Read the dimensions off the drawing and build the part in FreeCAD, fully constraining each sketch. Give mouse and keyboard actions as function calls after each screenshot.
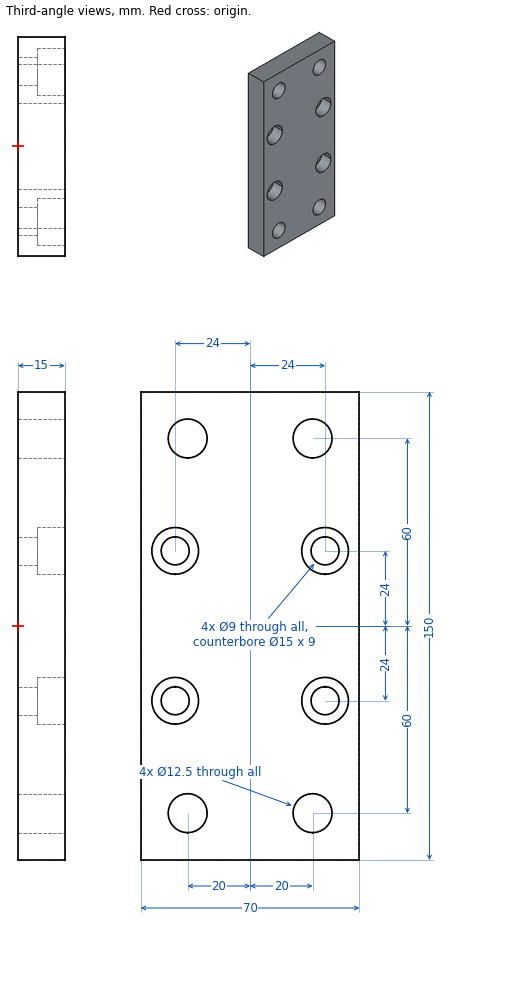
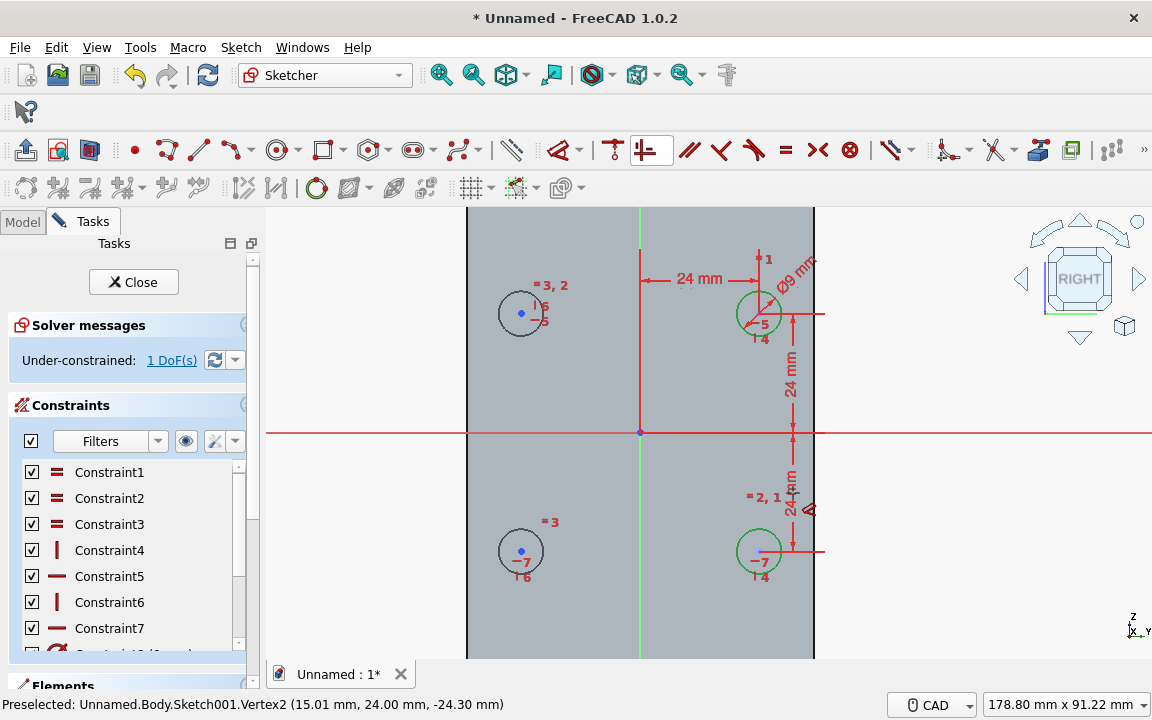
click(521, 314)
click(581, 280)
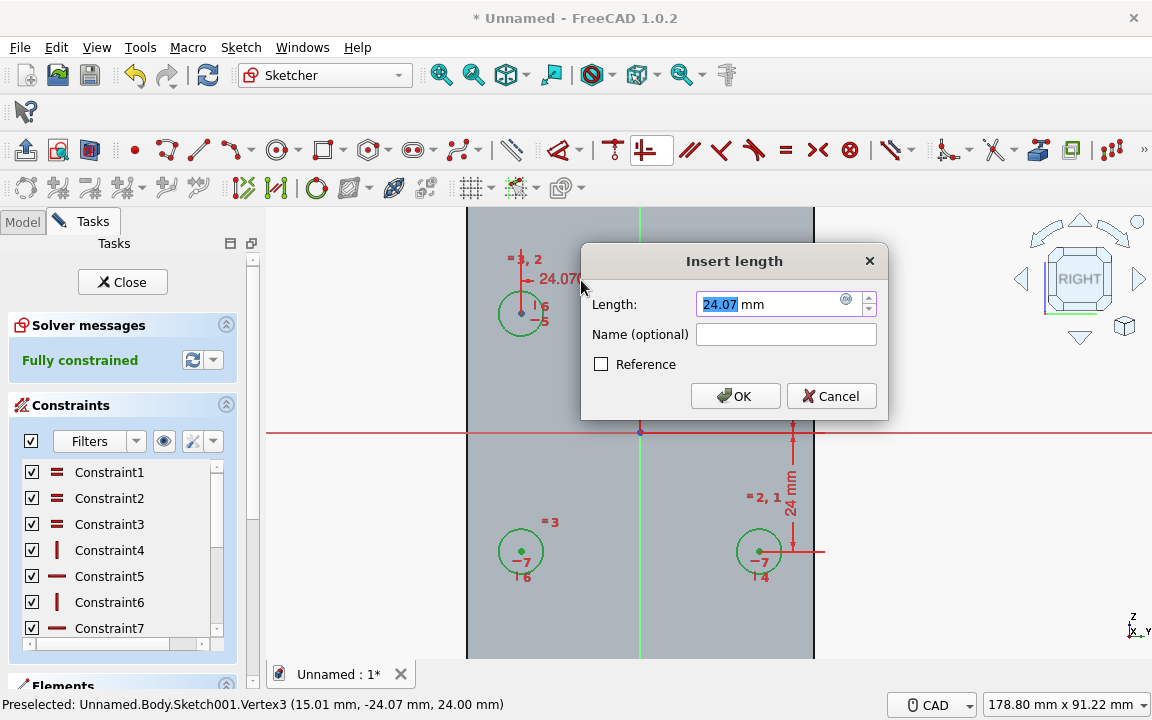
text(24)
key(Return)
key(Escape)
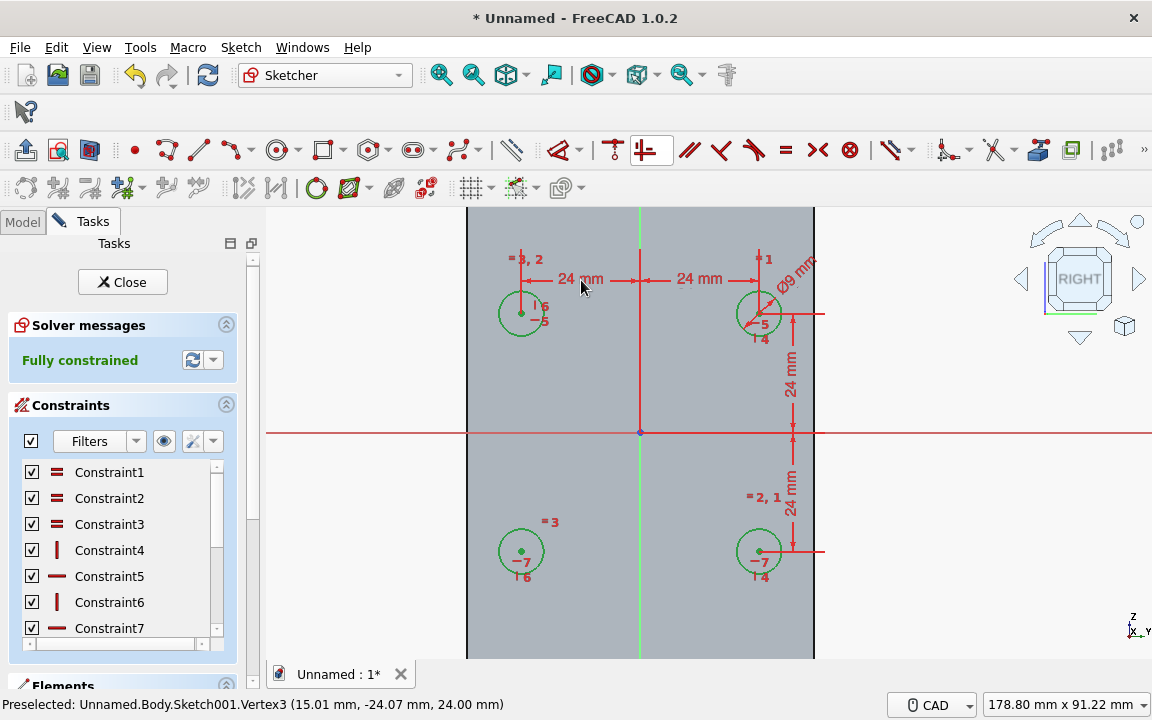
click(123, 282)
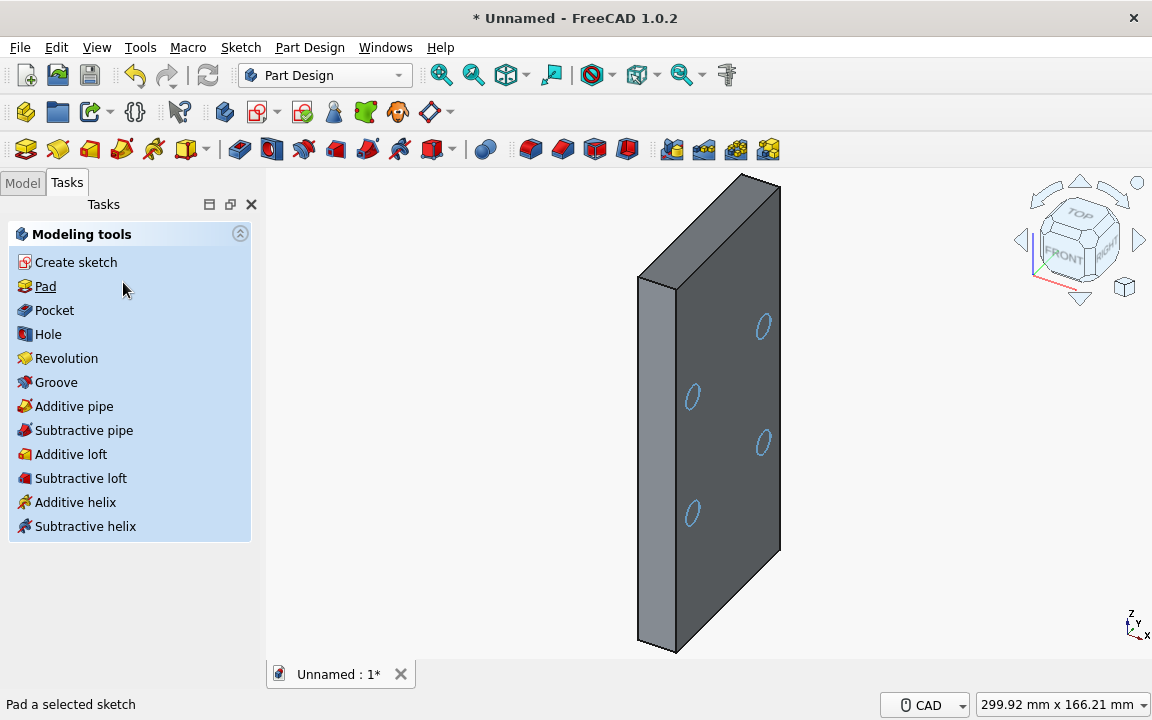
click(272, 150)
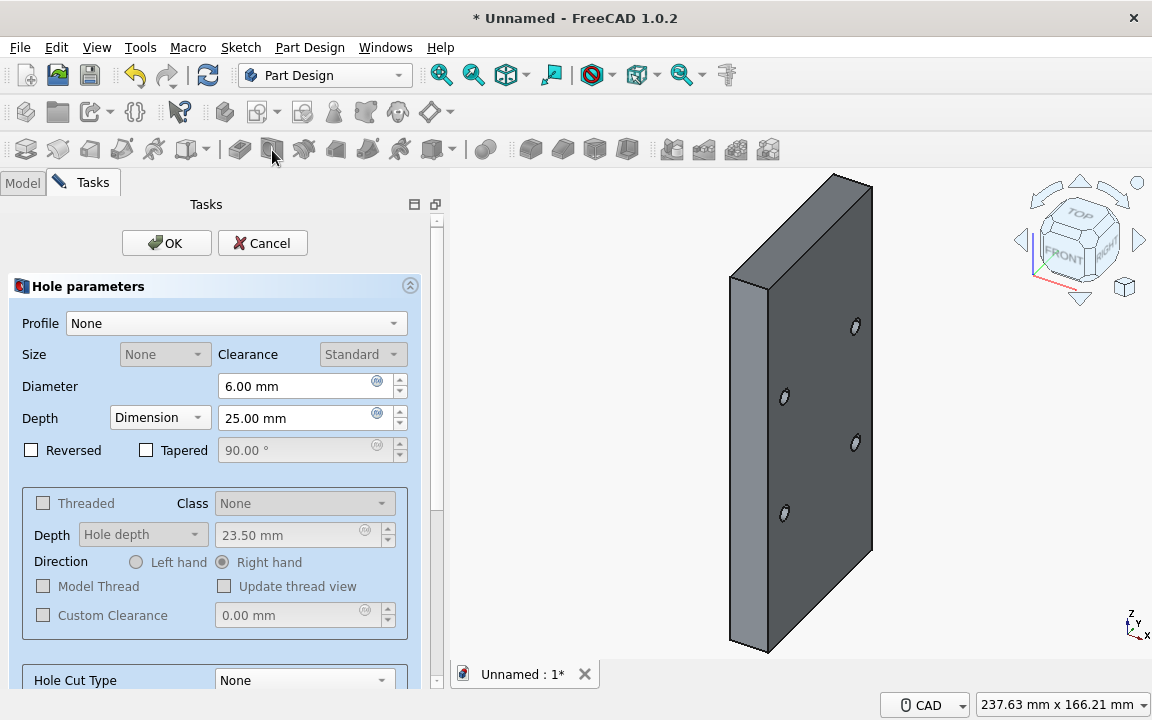
triple_click(305, 386)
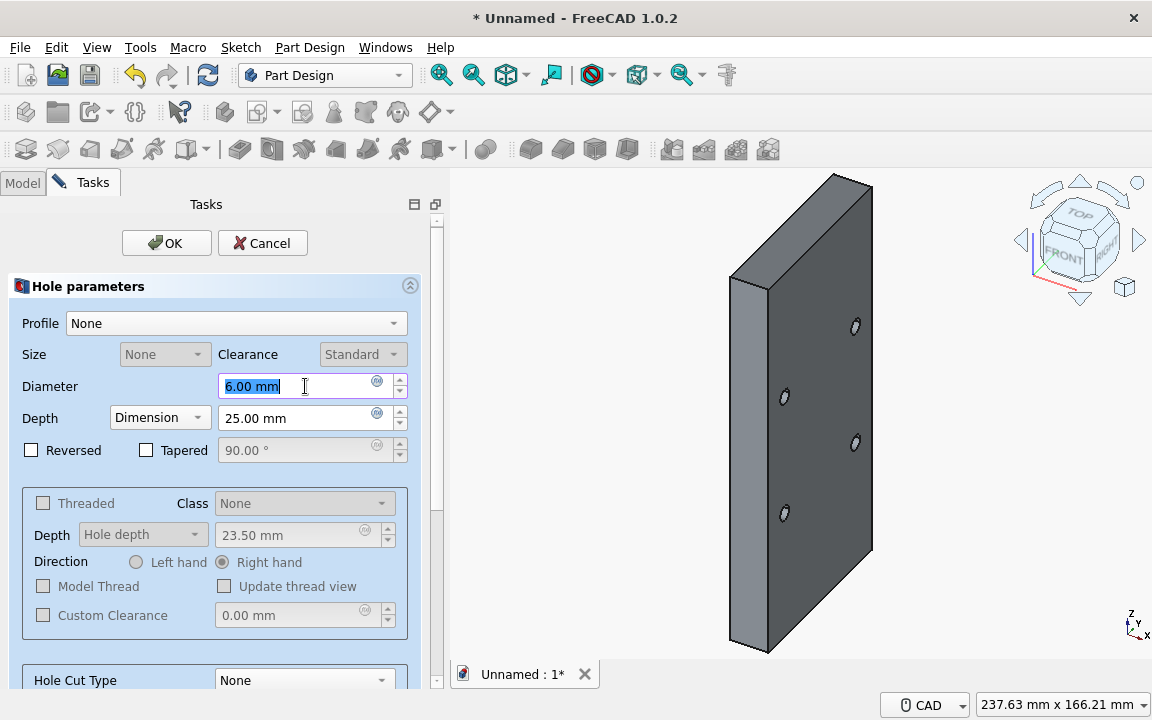
text(9)
key(Tab)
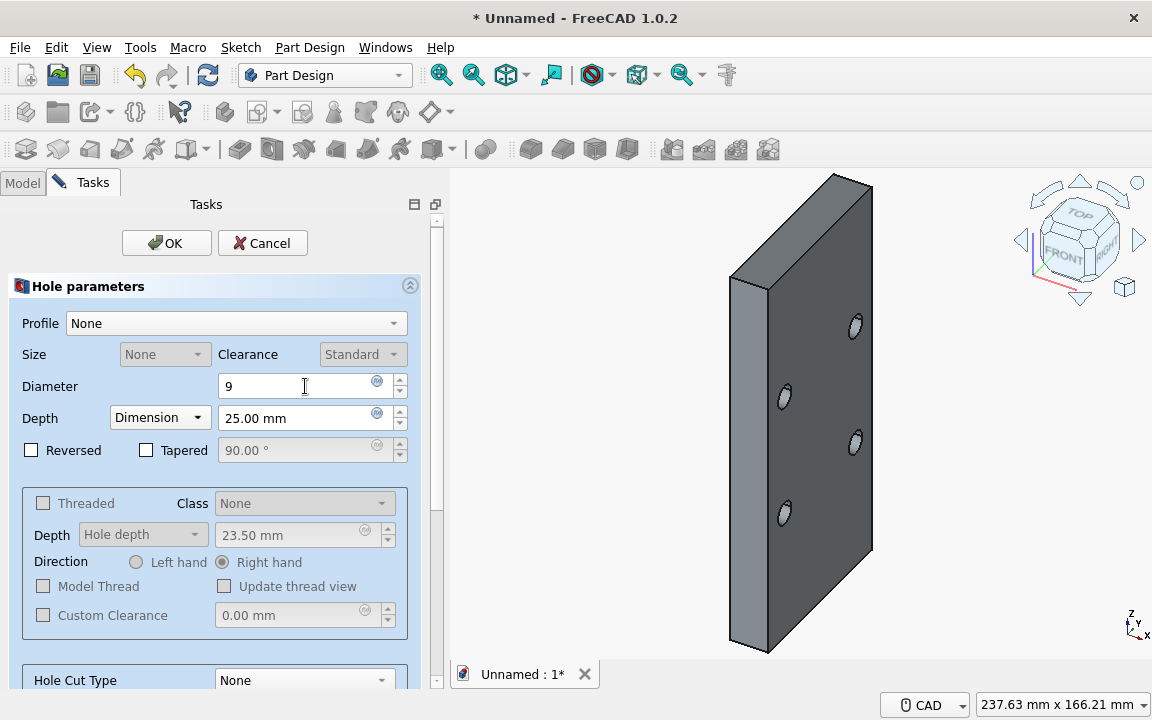
click(161, 418)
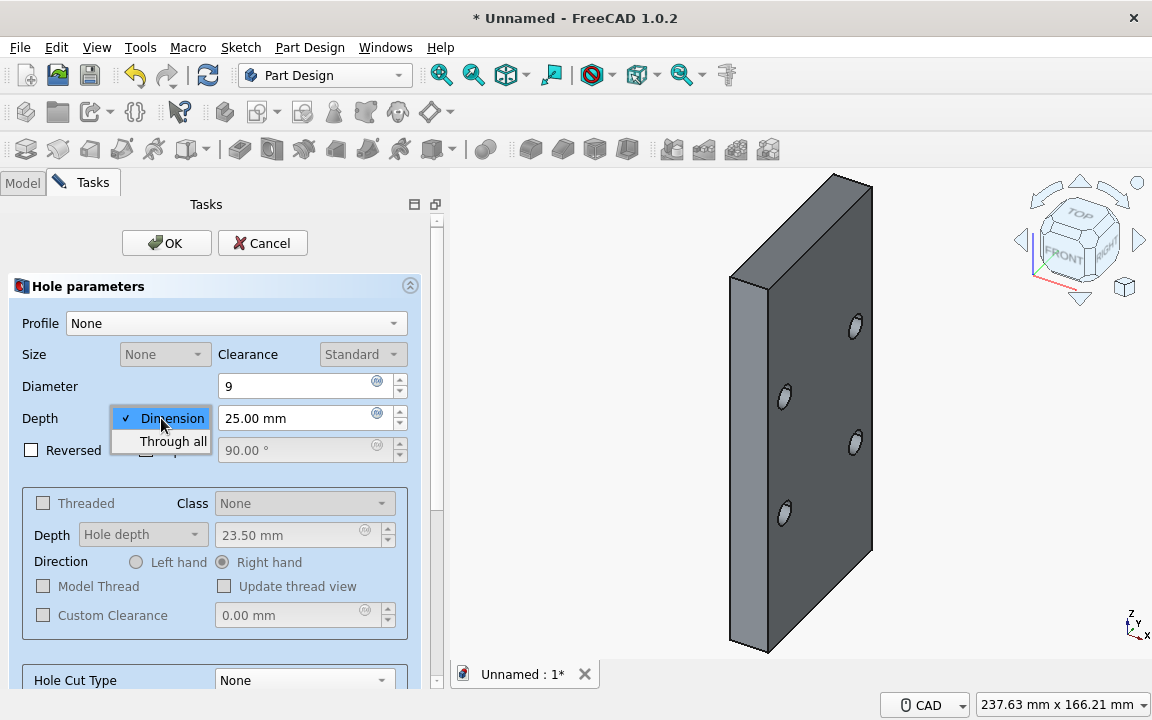
click(160, 442)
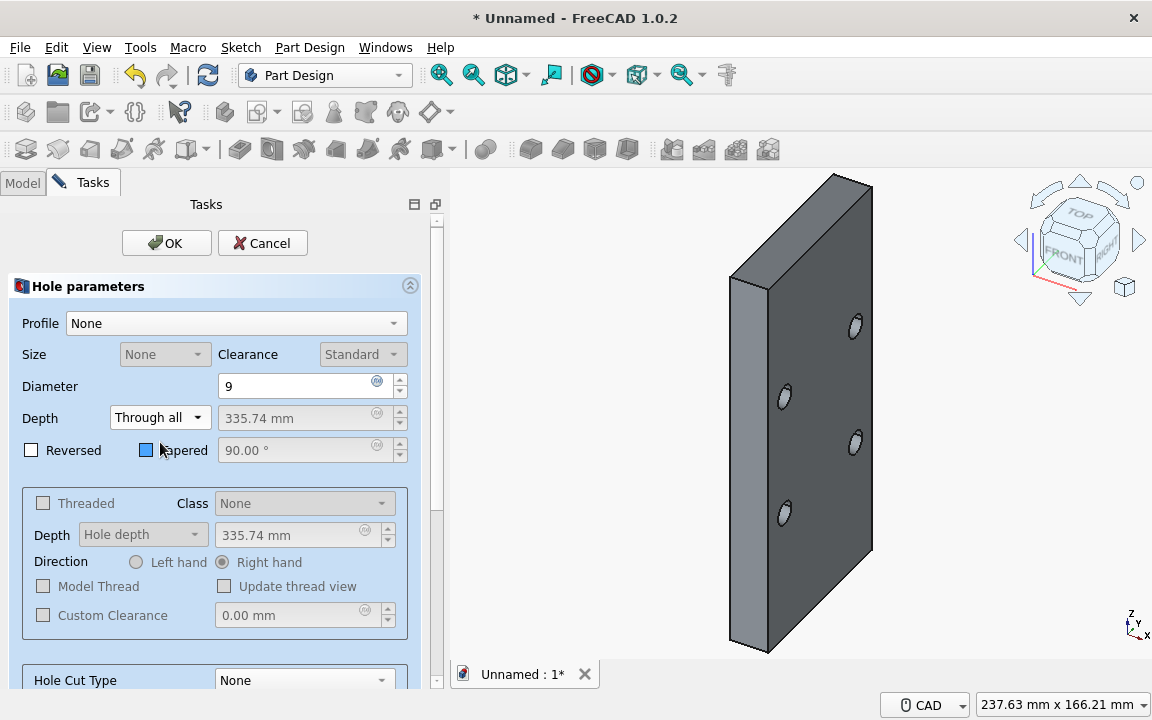
scroll(437, 451, down, 2)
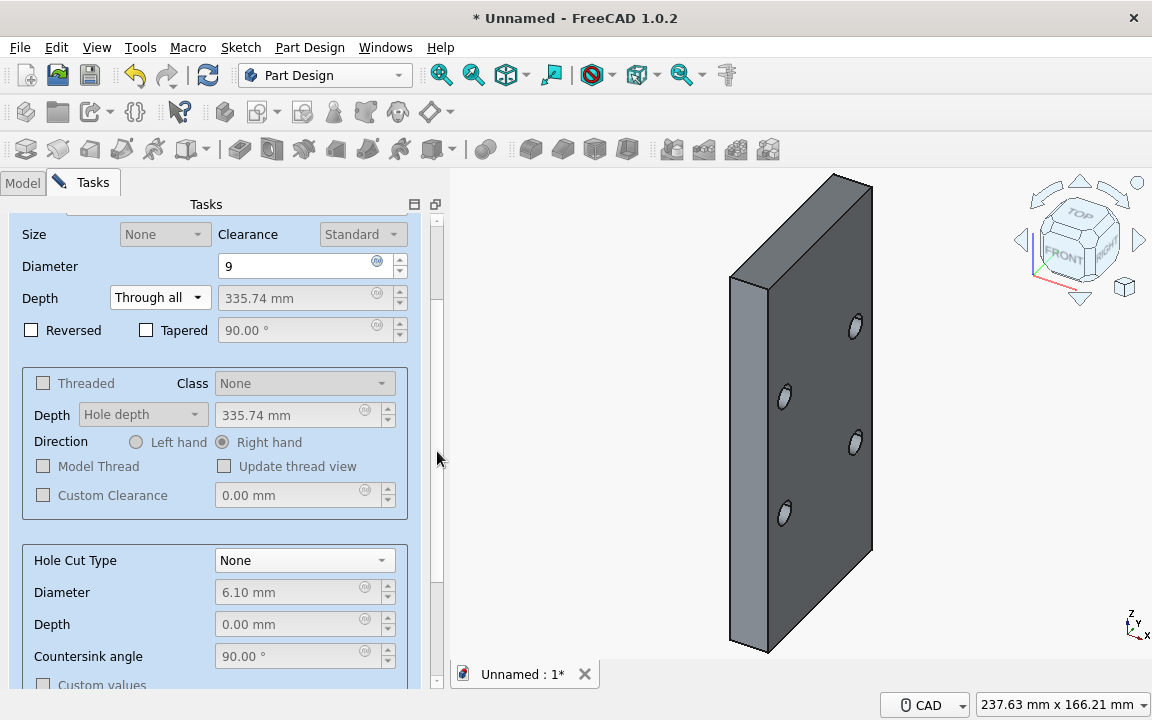
click(306, 560)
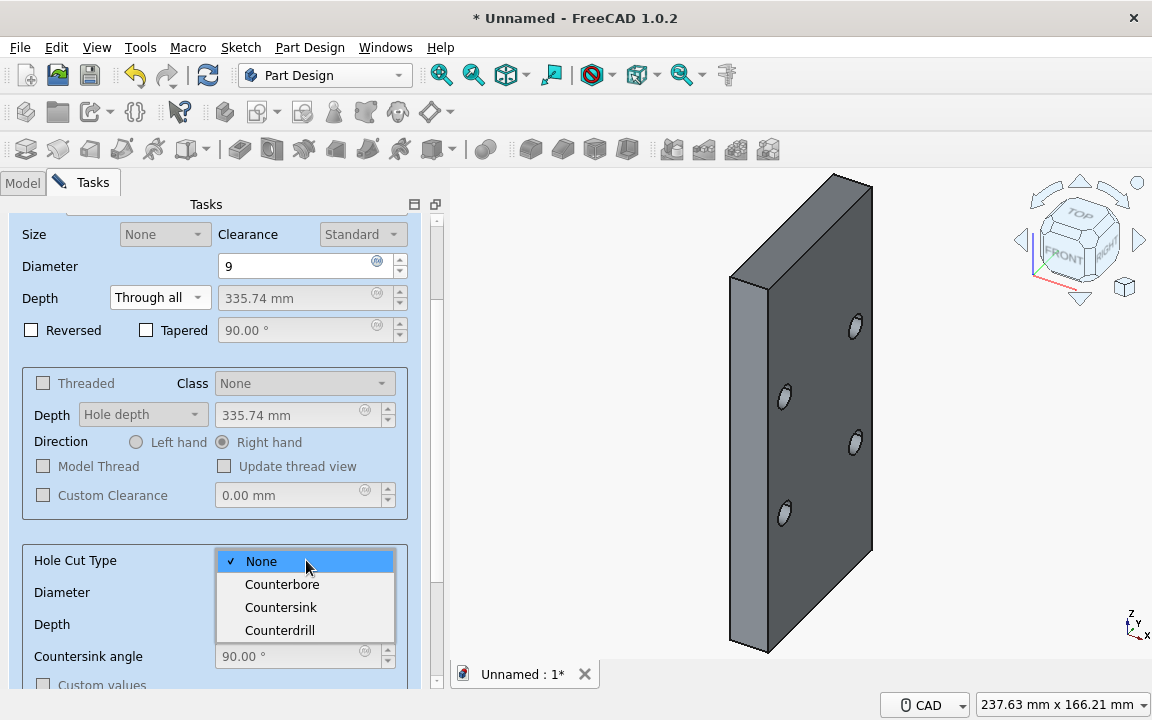
click(304, 584)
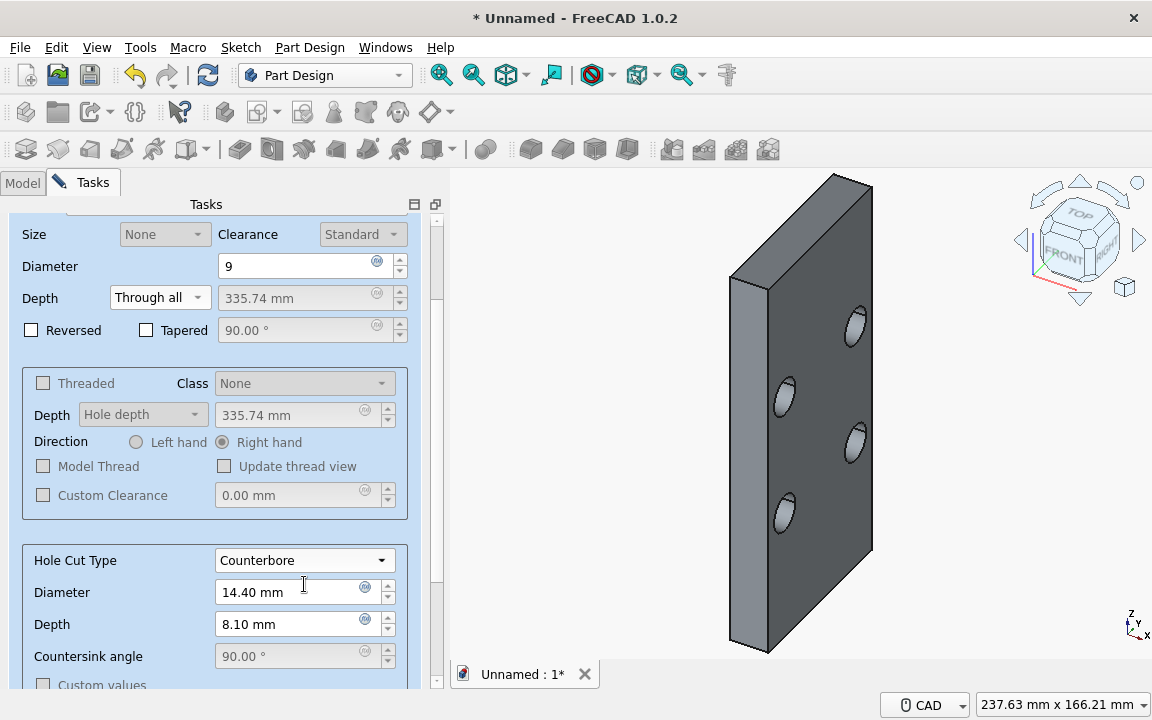
triple_click(298, 592)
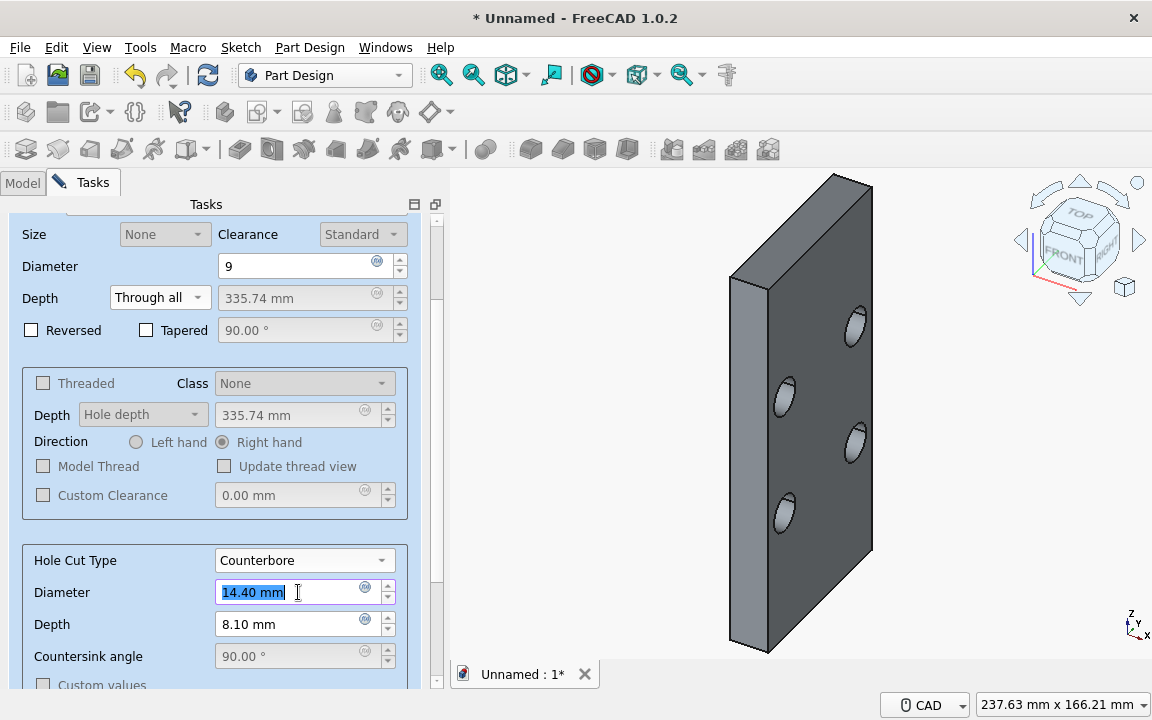
text(15)
key(Tab)